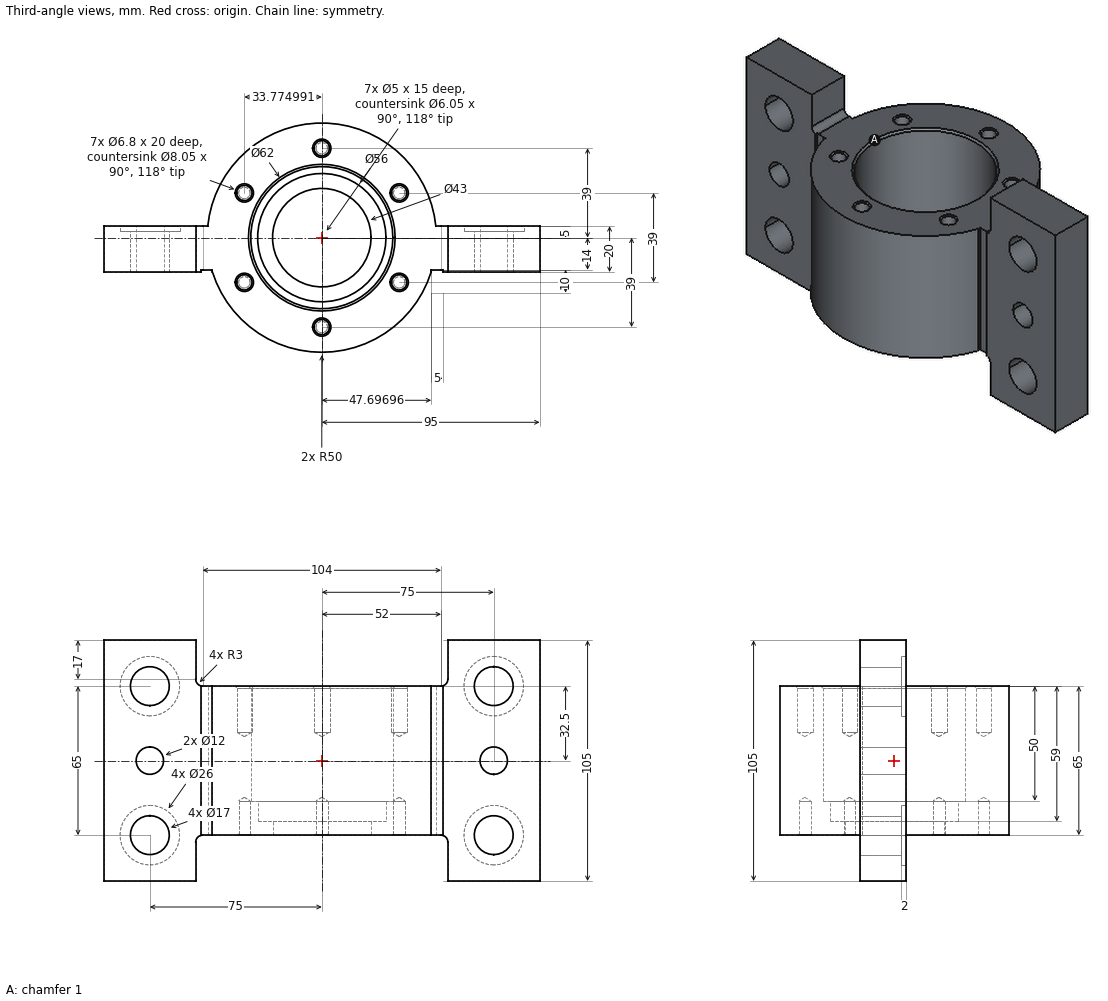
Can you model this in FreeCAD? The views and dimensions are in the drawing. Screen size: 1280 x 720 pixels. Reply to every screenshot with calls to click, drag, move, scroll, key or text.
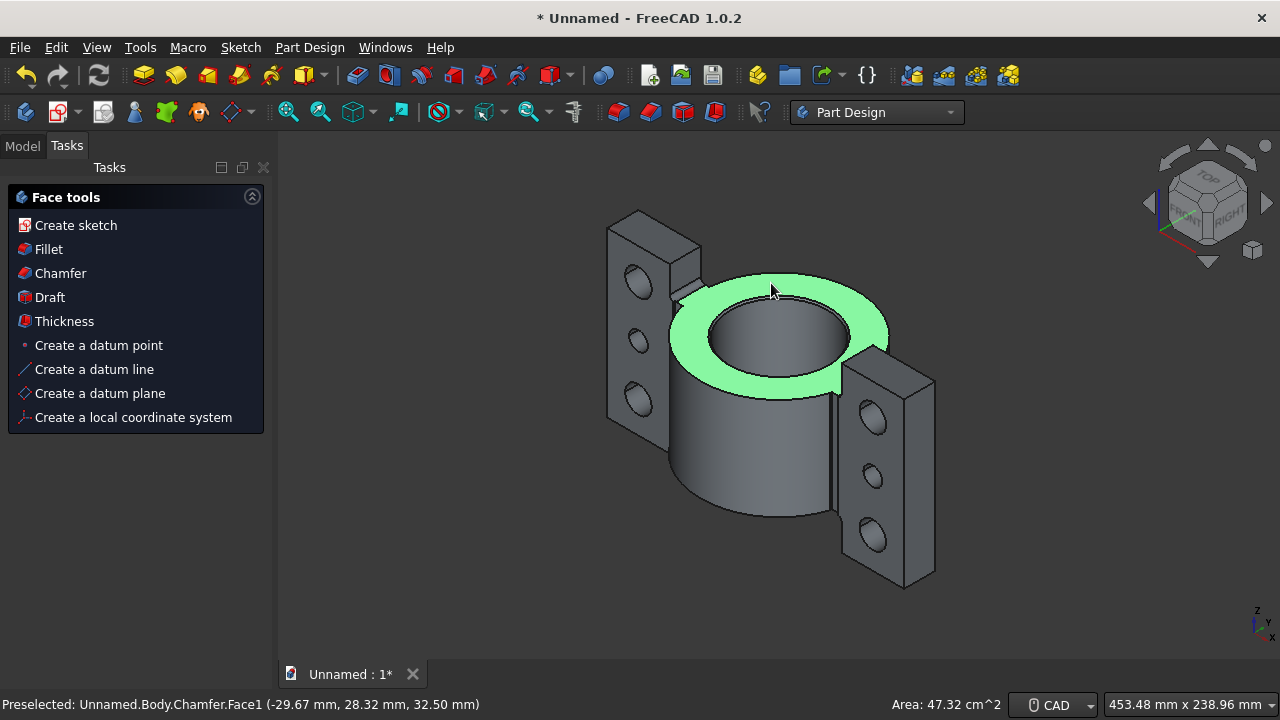
click(58, 112)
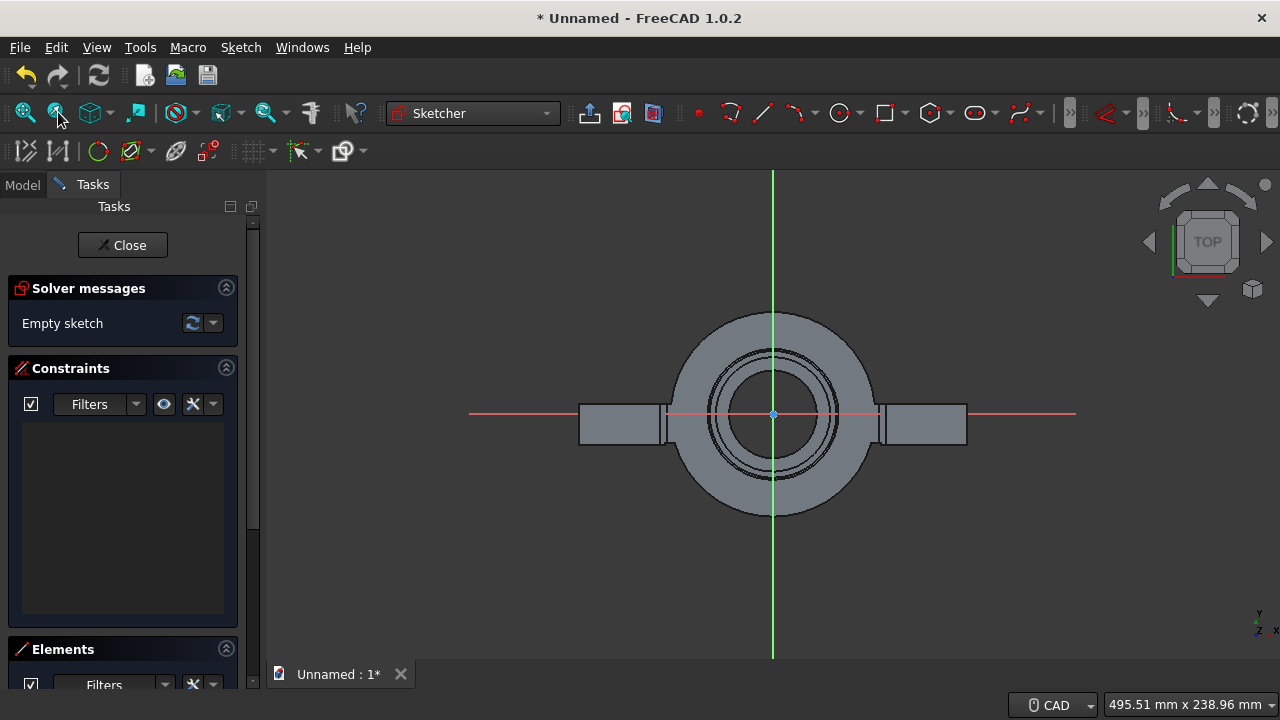
scroll(856, 414, up, 3)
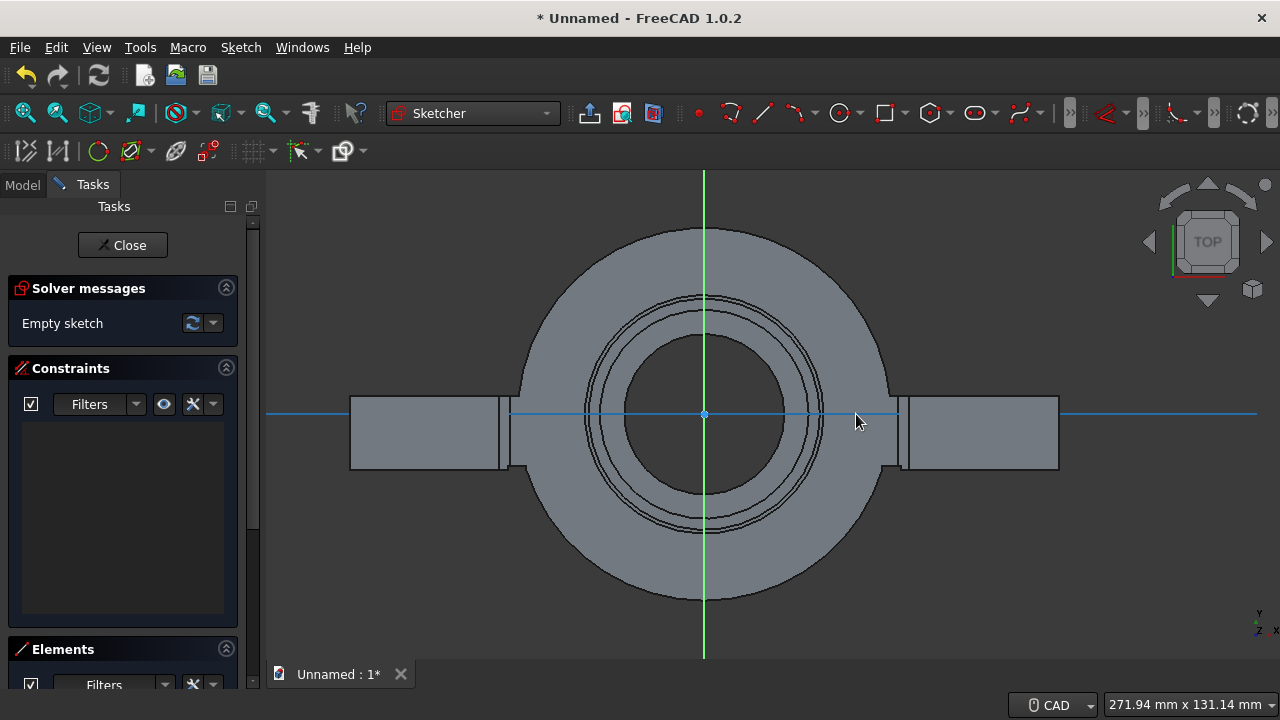
click(840, 114)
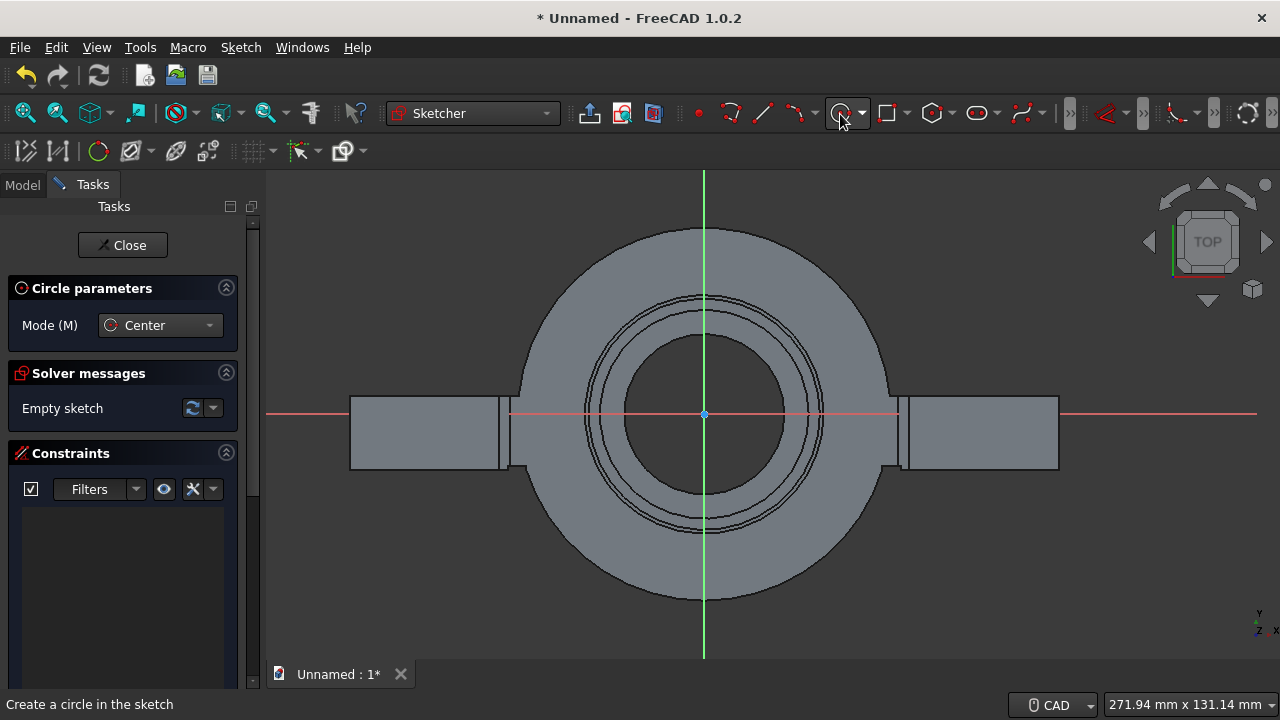
scroll(578, 342, up, 3)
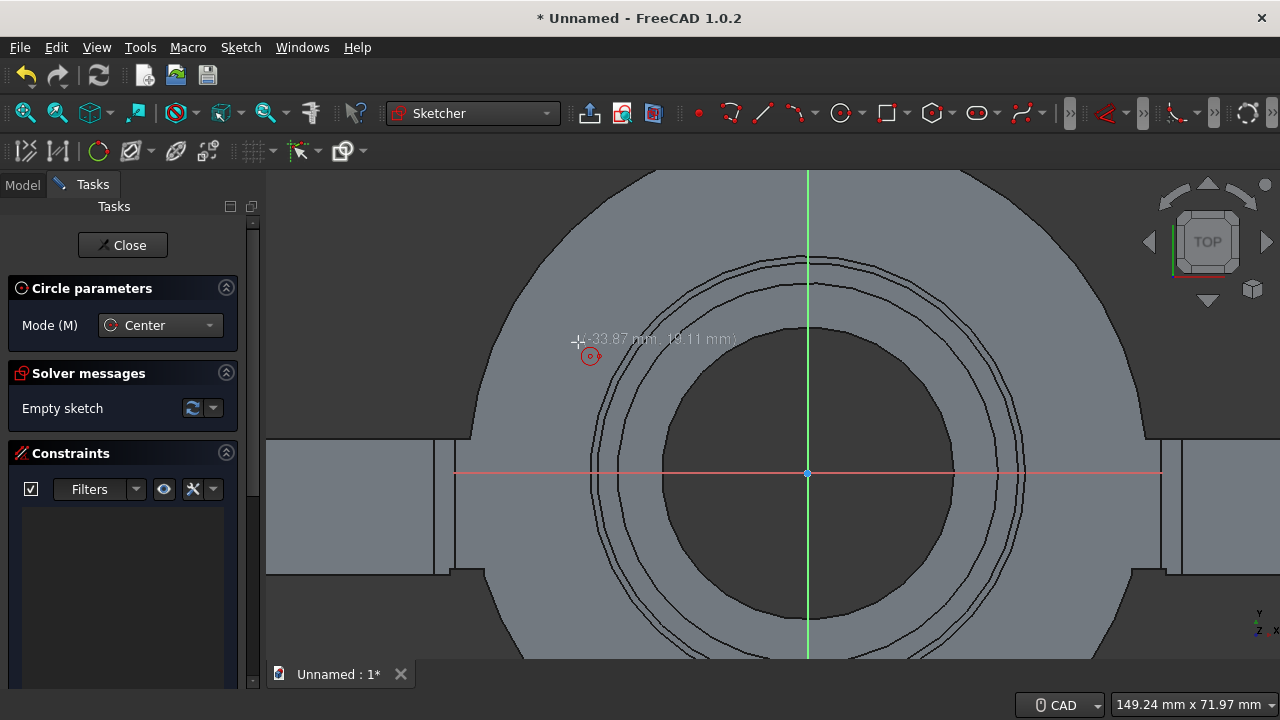
click(578, 341)
click(595, 325)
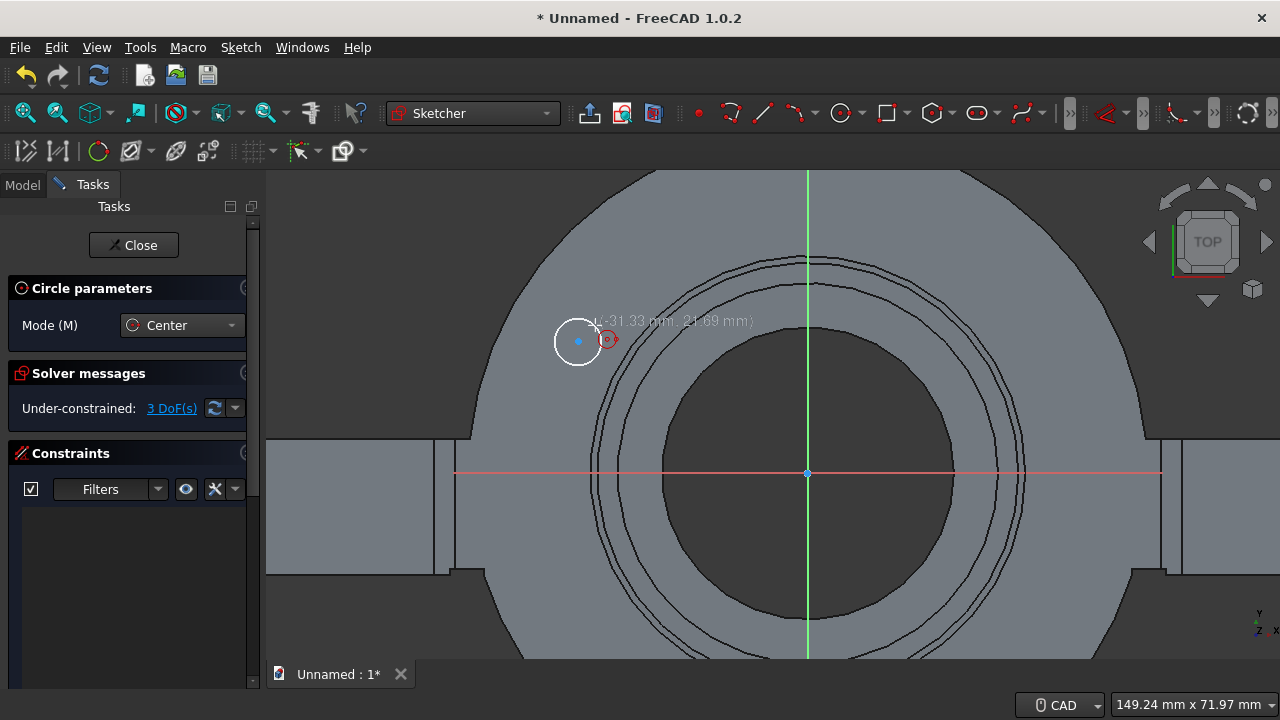
click(808, 208)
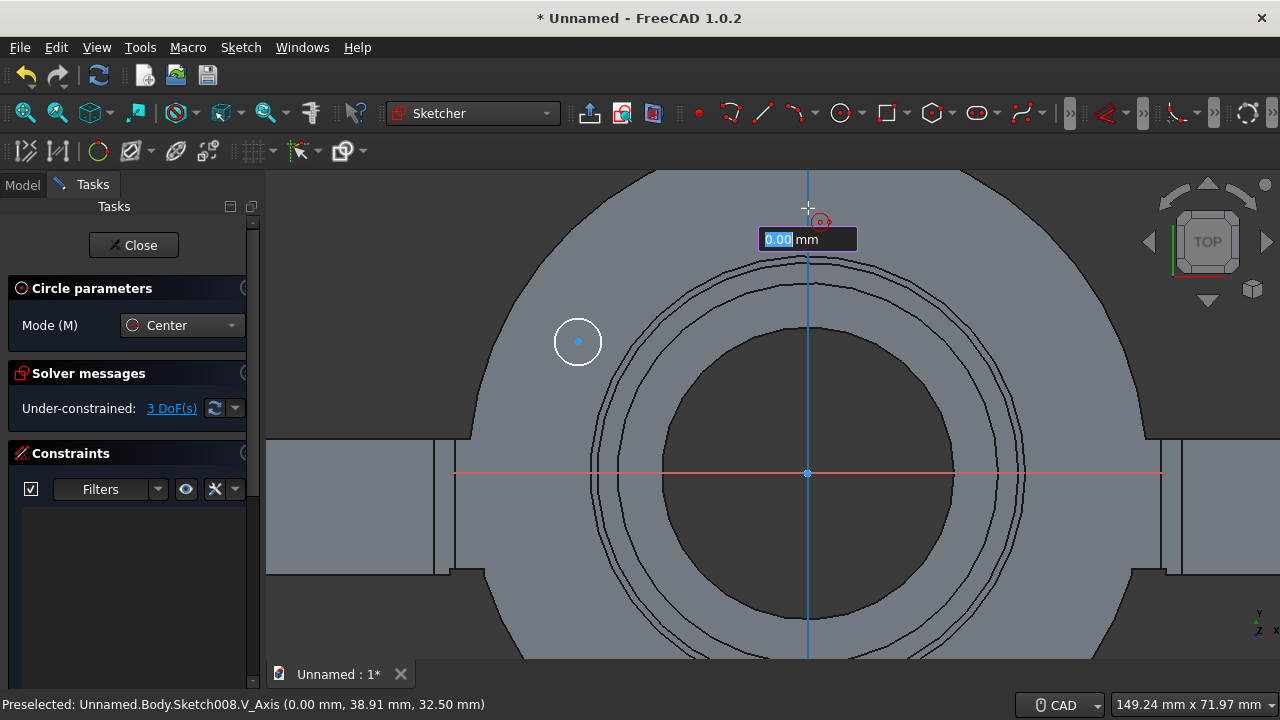
scroll(579, 343, down, 3)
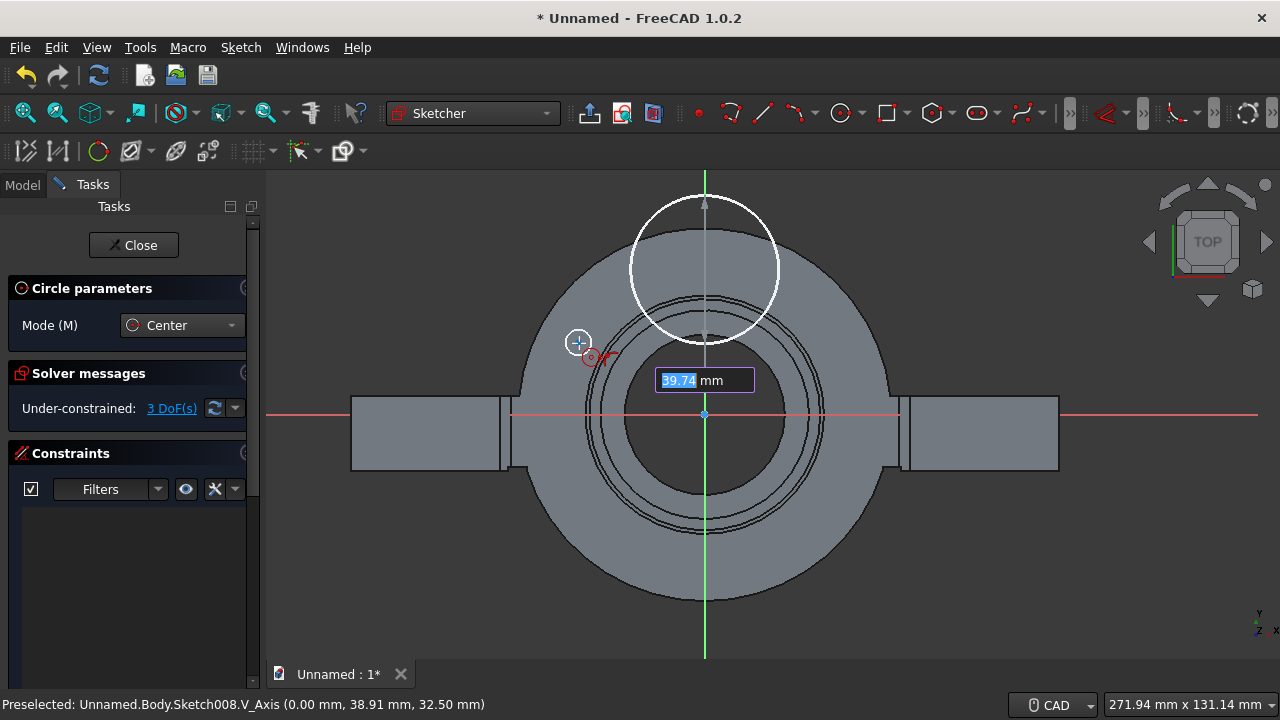
scroll(714, 260, up, 3)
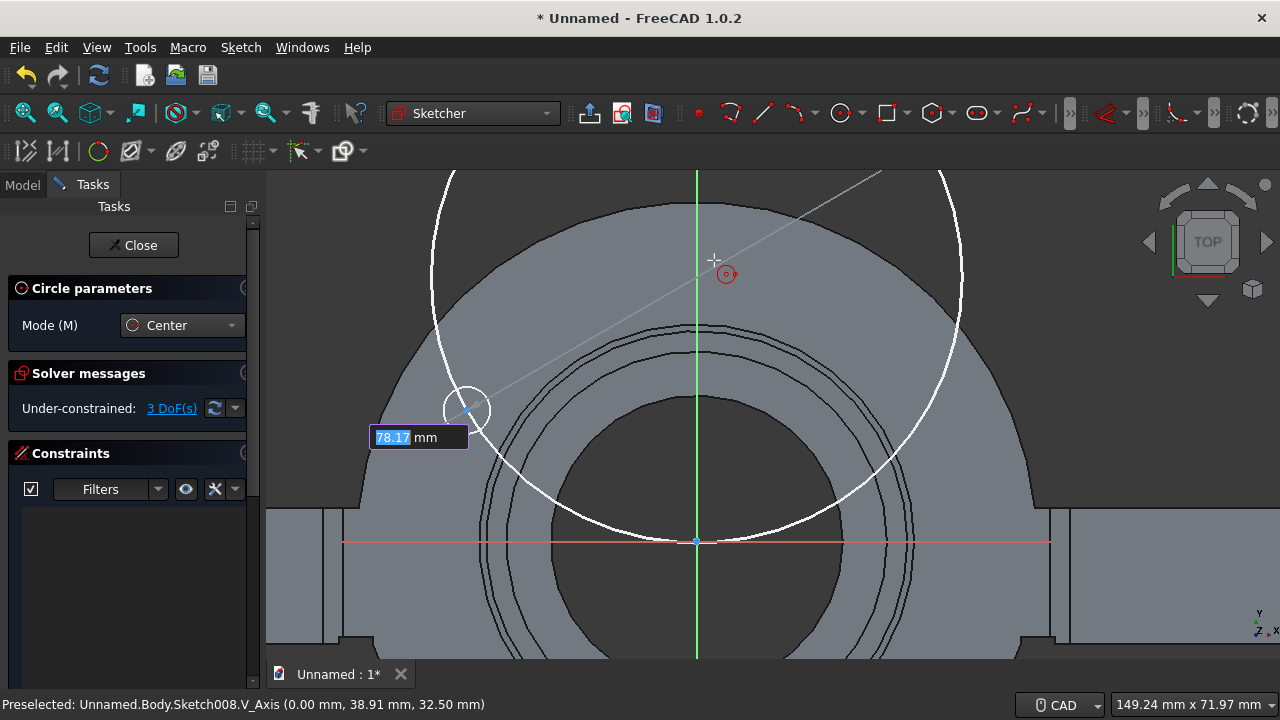
click(713, 260)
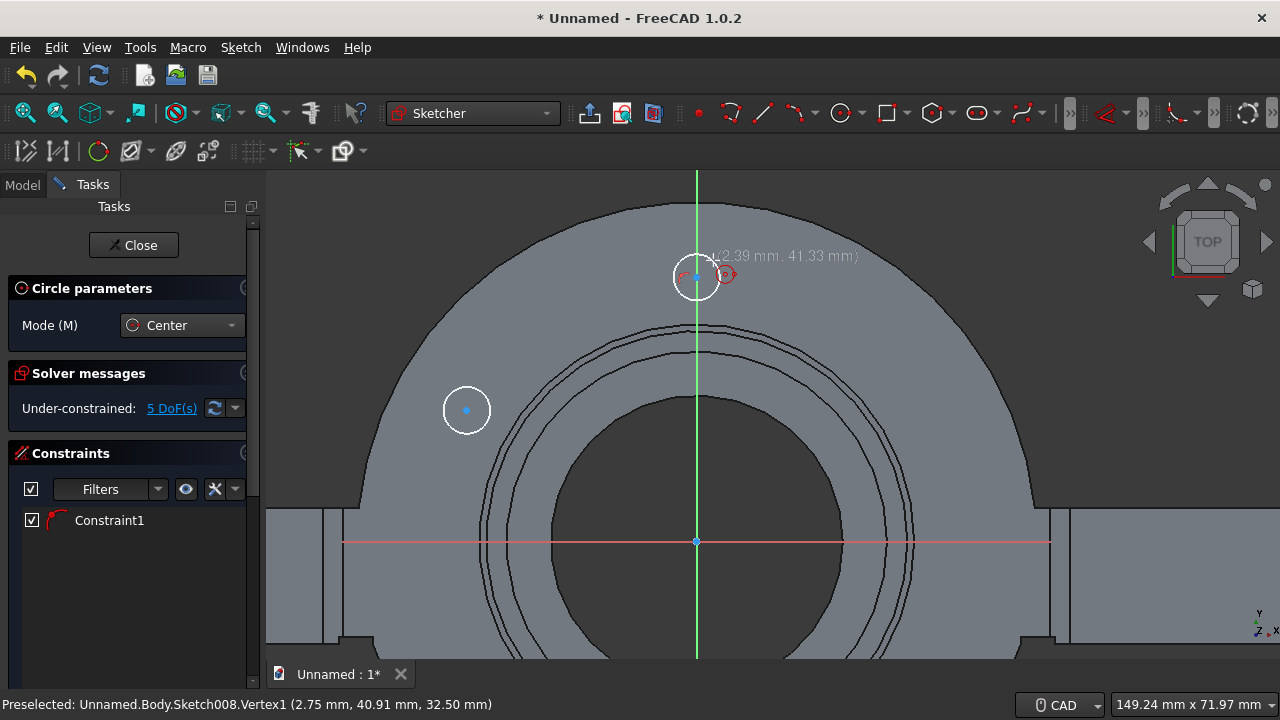
click(926, 409)
click(943, 393)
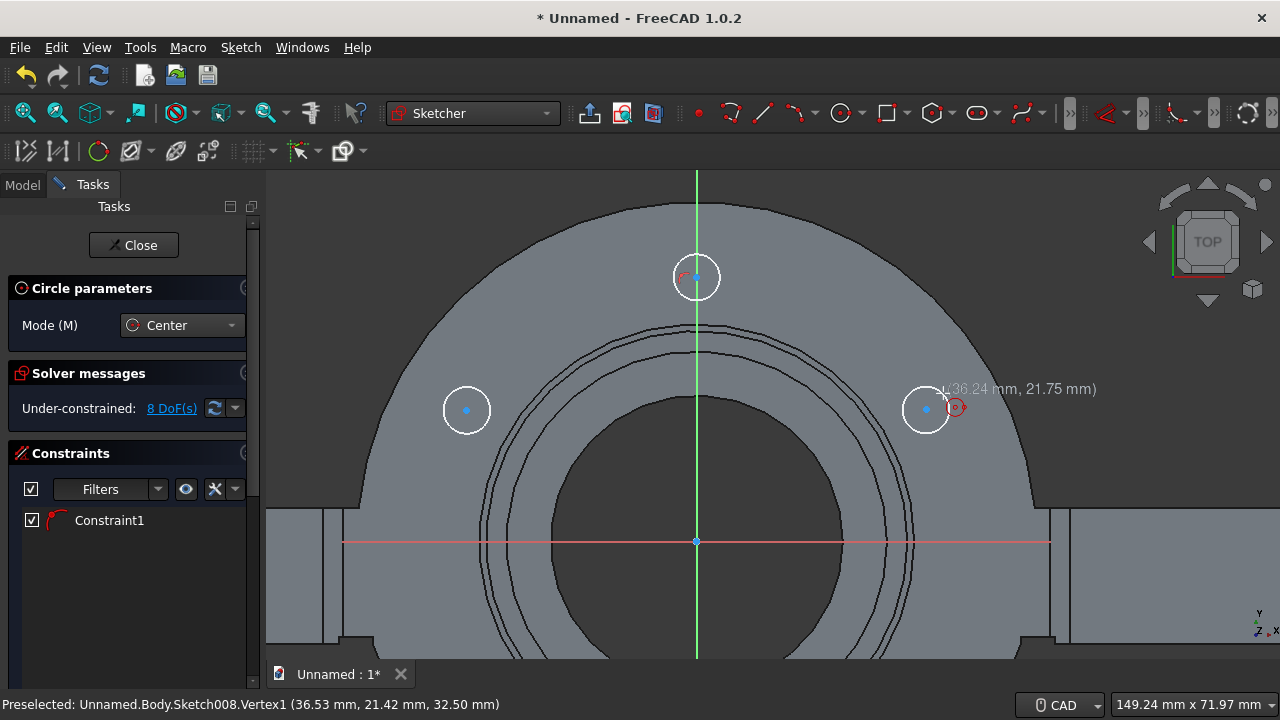
scroll(714, 260, down, 3)